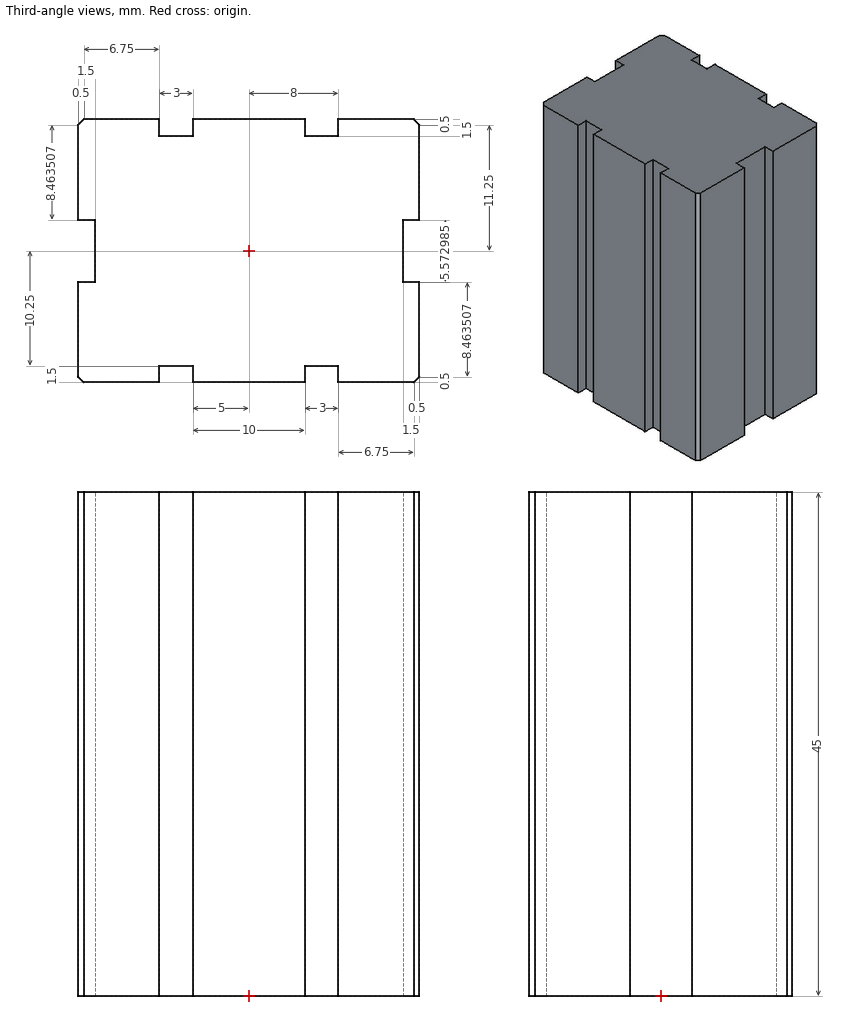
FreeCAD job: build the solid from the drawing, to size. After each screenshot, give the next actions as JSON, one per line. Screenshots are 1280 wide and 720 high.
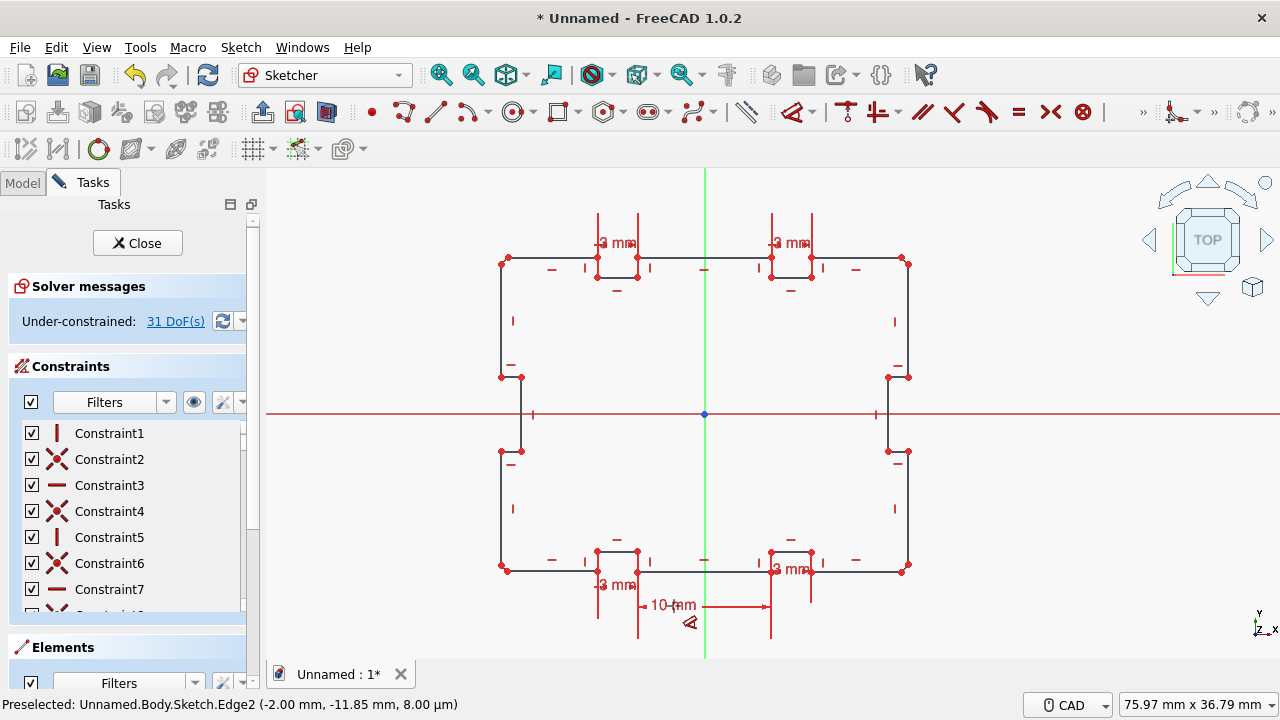
{"action": "left_click", "coordinate": [731, 258]}
{"action": "left_click", "coordinate": [674, 224]}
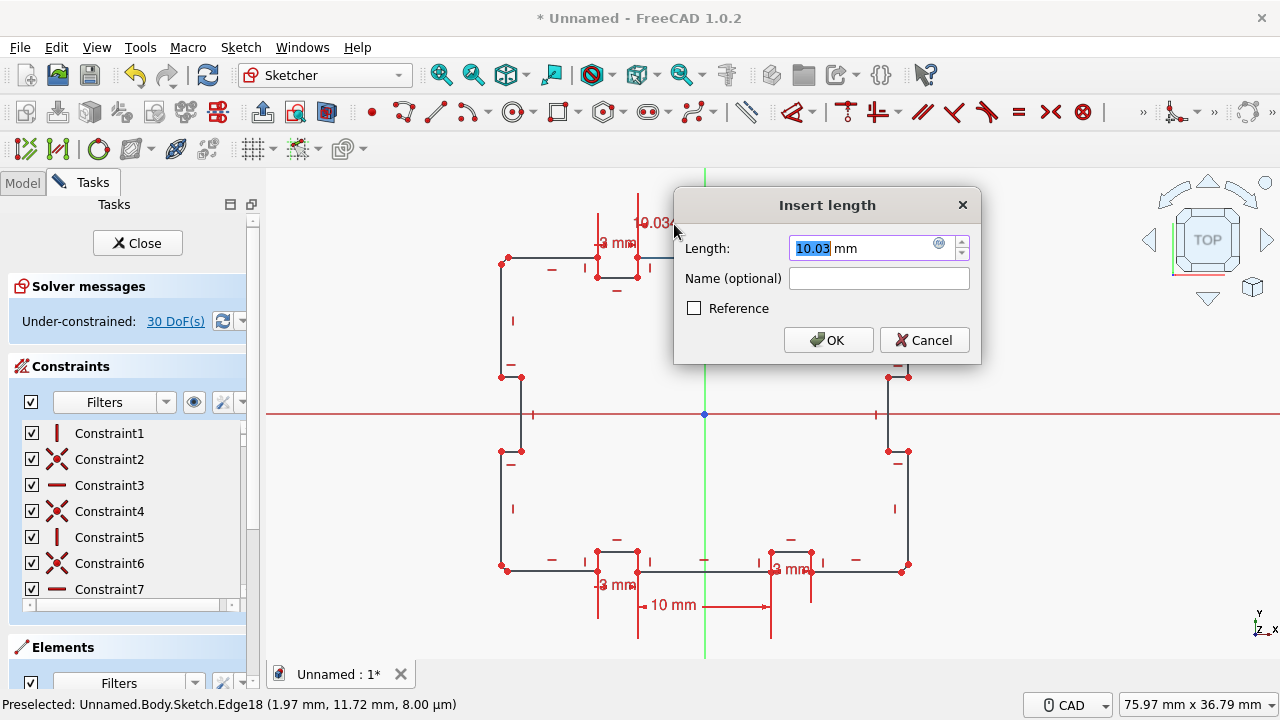
{"action": "type", "text": "10"}
{"action": "key", "text": "Return"}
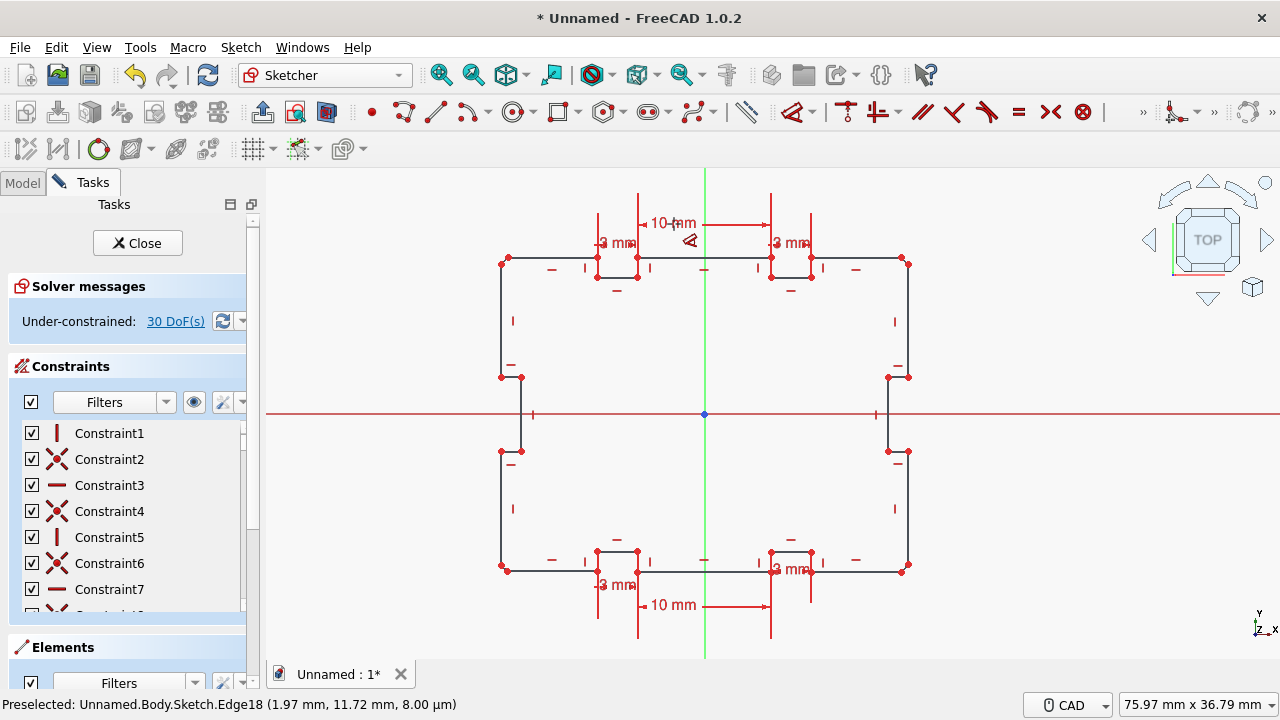
{"action": "left_click", "coordinate": [638, 552]}
{"action": "left_click", "coordinate": [671, 380]}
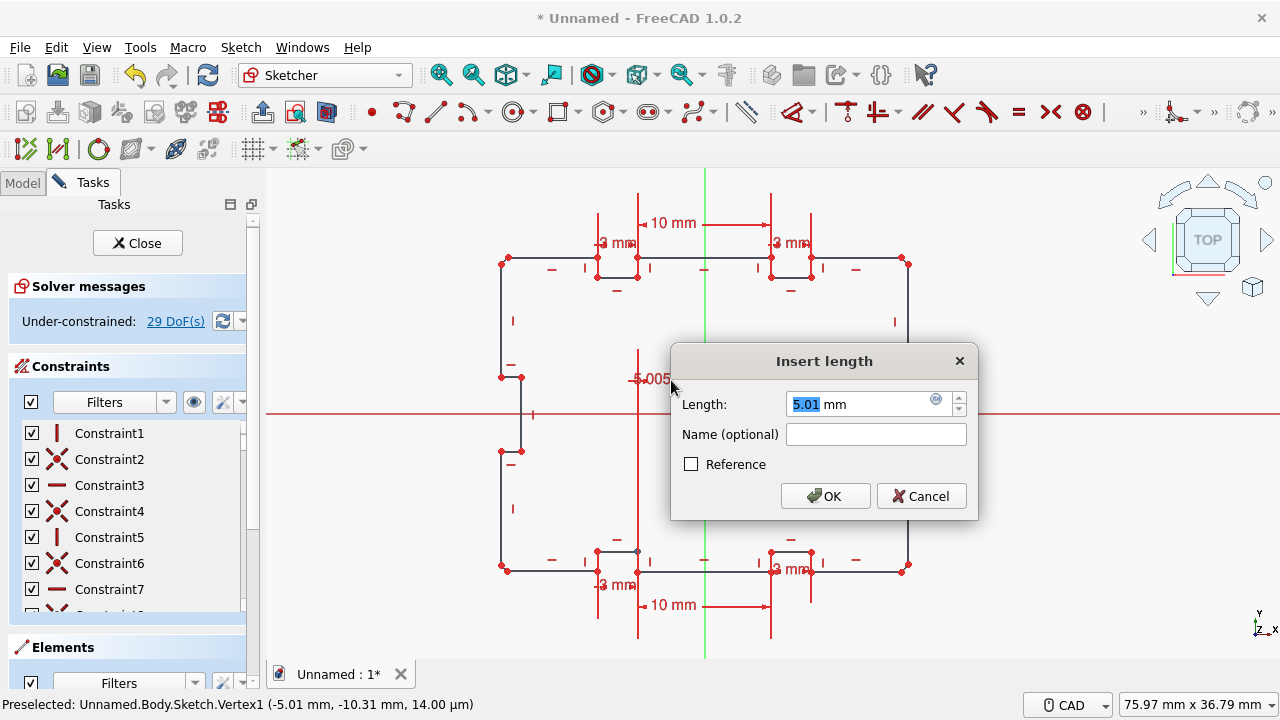
{"action": "type", "text": "5"}
{"action": "key", "text": "Return"}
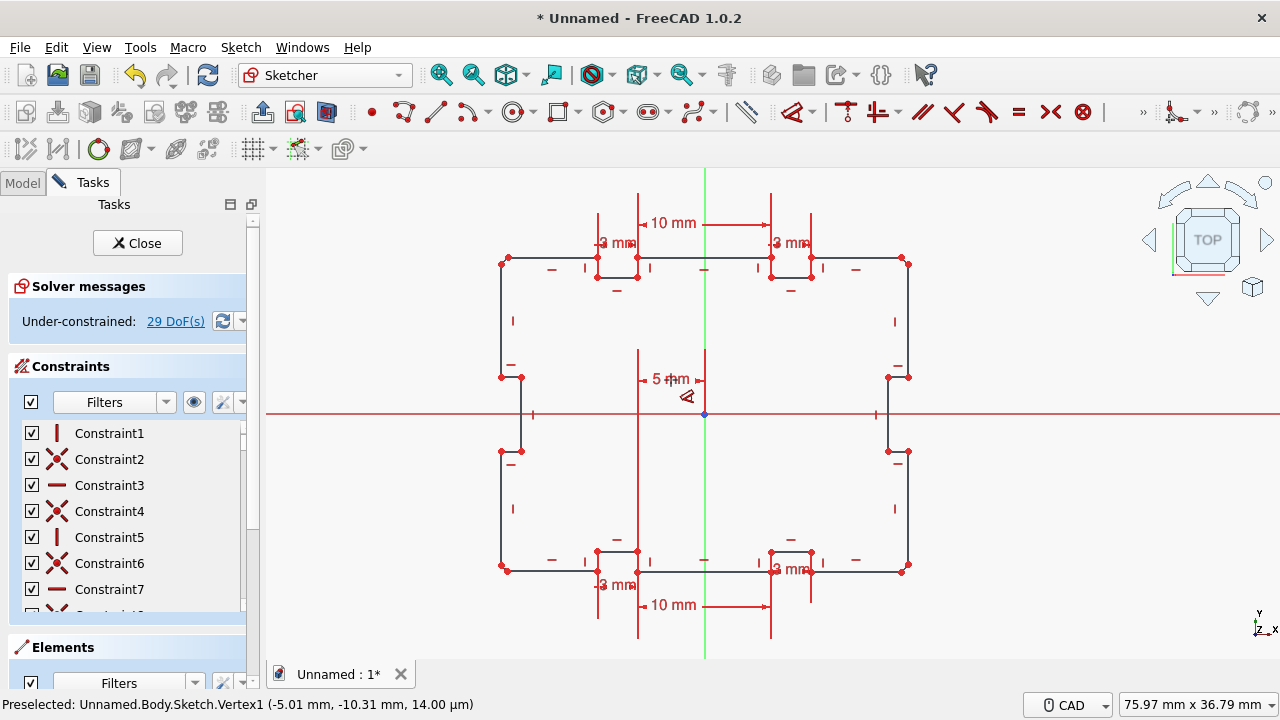
{"action": "left_click", "coordinate": [811, 258]}
{"action": "left_click", "coordinate": [758, 224]}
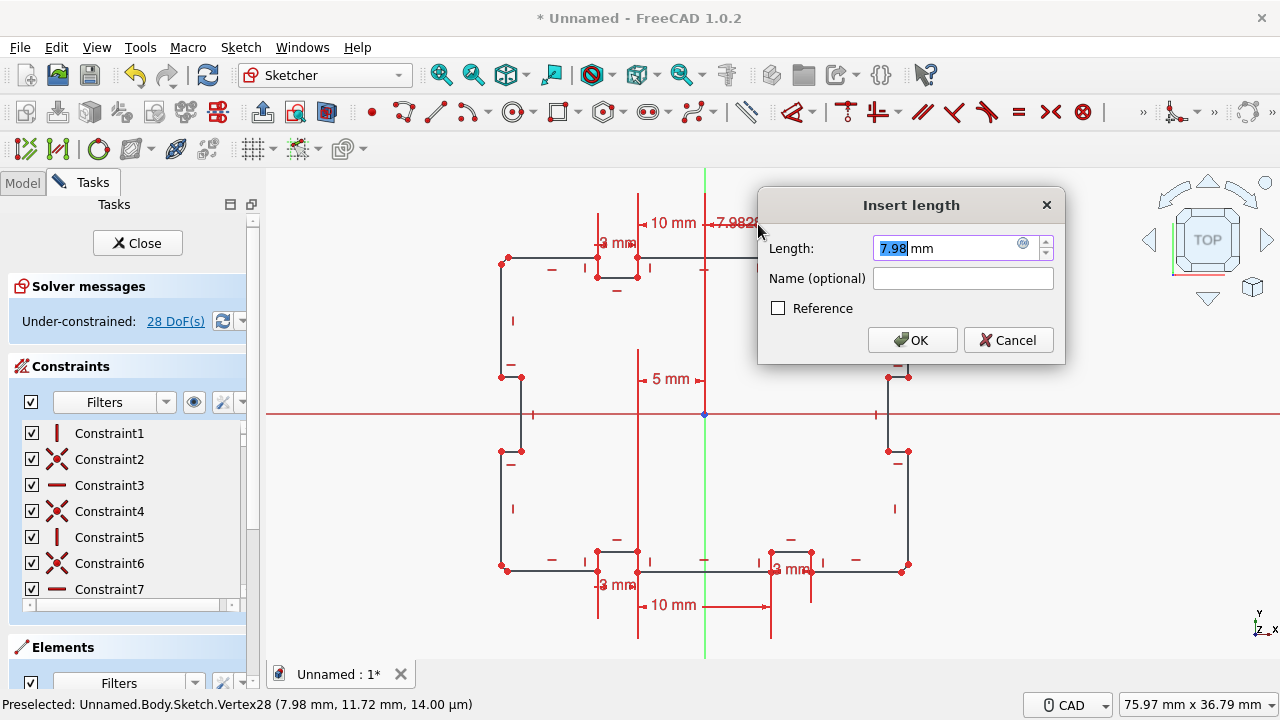
{"action": "type", "text": "8"}
{"action": "key", "text": "Return"}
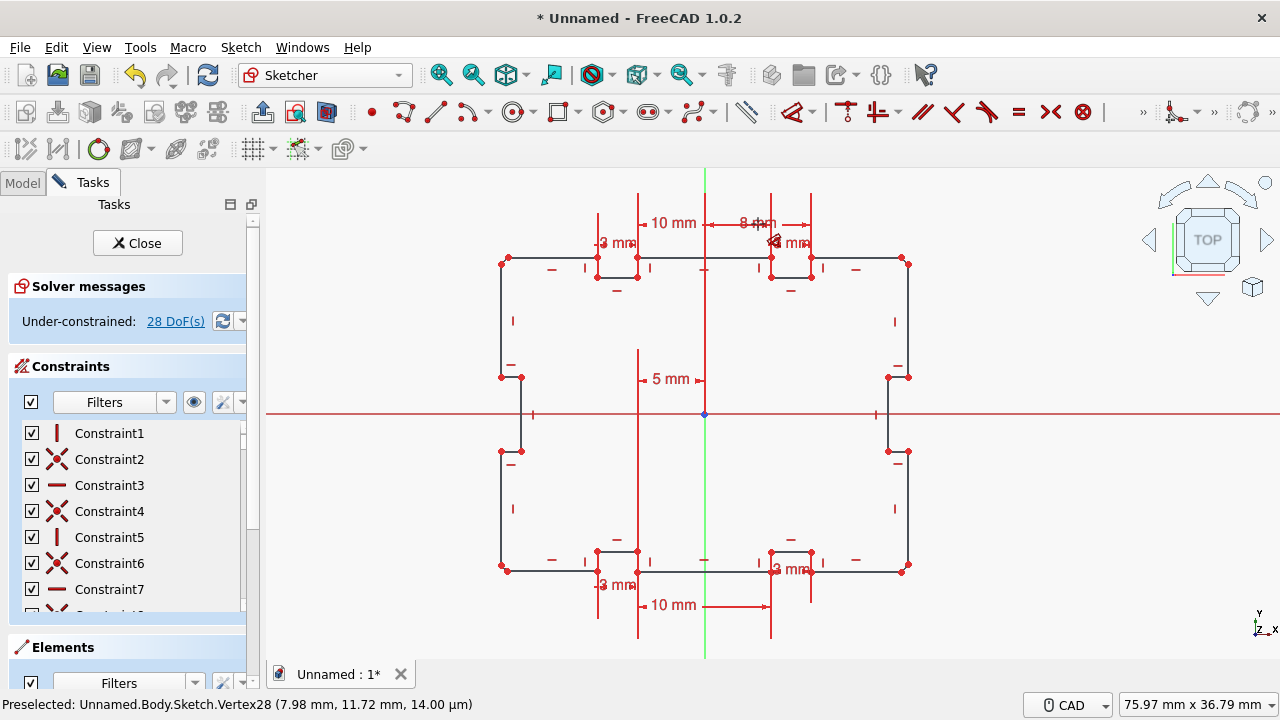
{"action": "scroll", "coordinate": [638, 562], "scroll_direction": "up", "scroll_amount": 4}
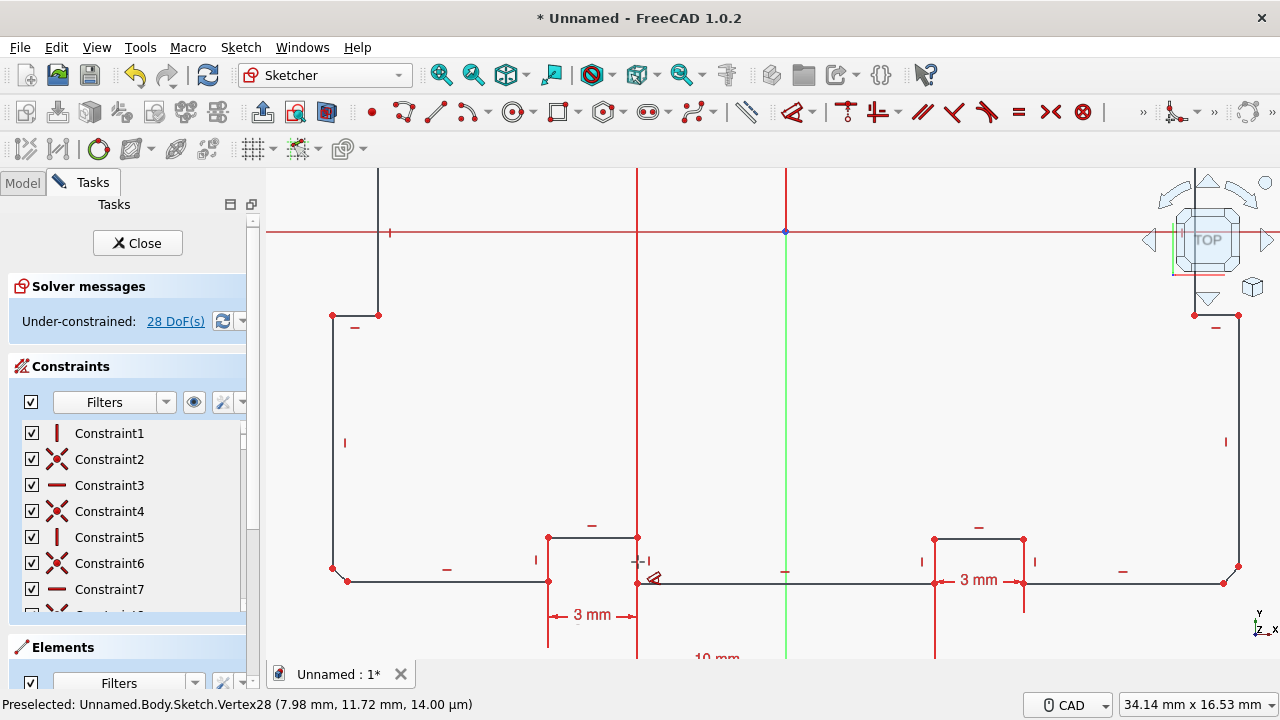
{"action": "left_click", "coordinate": [637, 561]}
{"action": "left_click", "coordinate": [603, 561]}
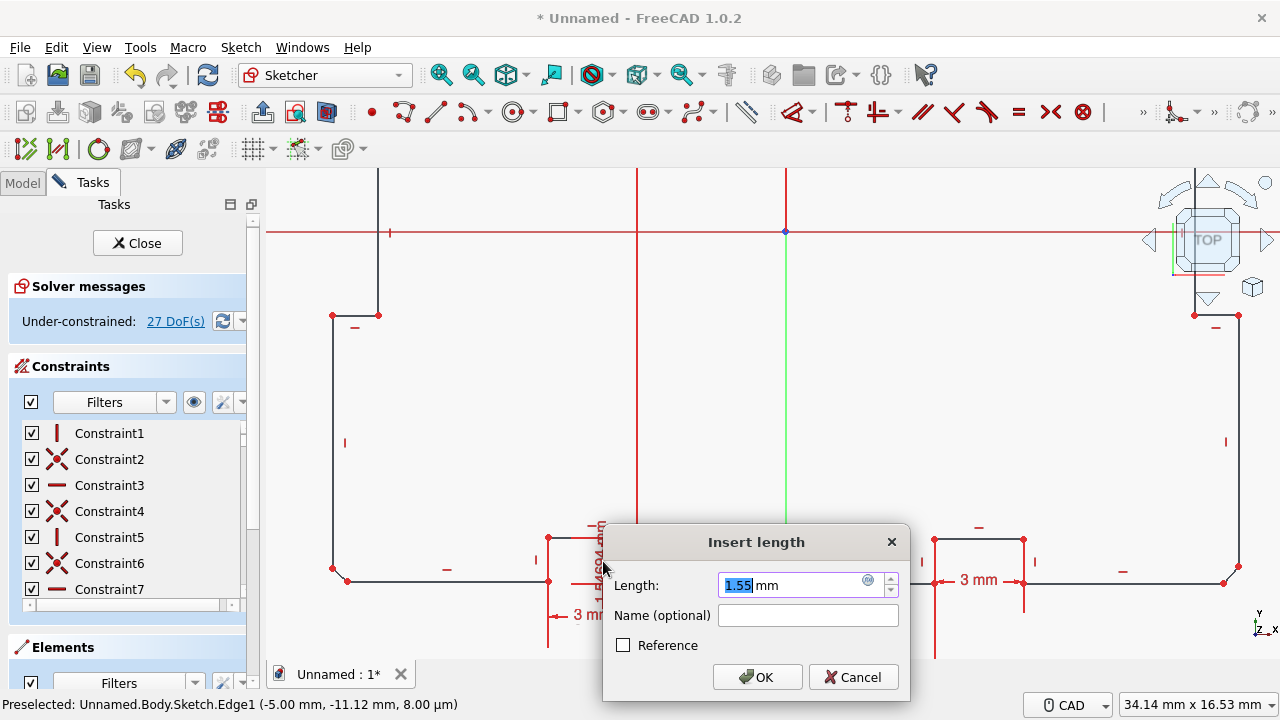
{"action": "type", "text": "1.5"}
{"action": "key", "text": "Return"}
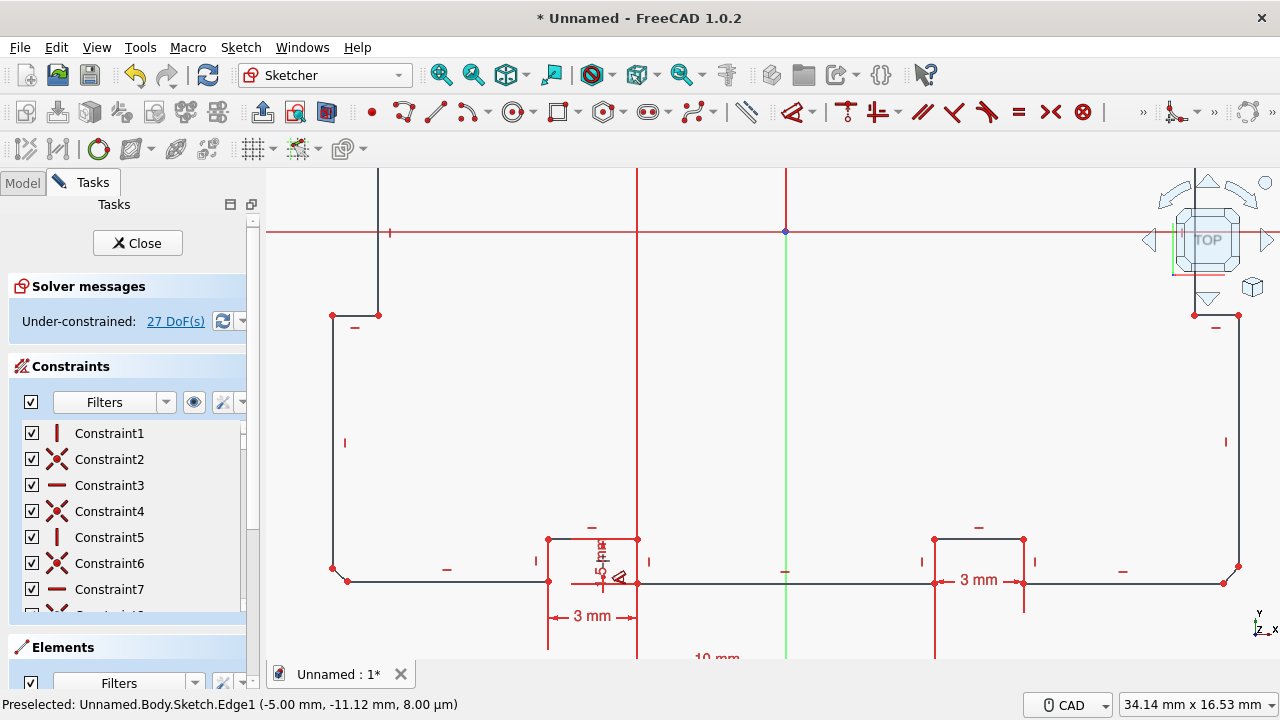
{"action": "left_click", "coordinate": [935, 570]}
{"action": "left_click", "coordinate": [901, 562]}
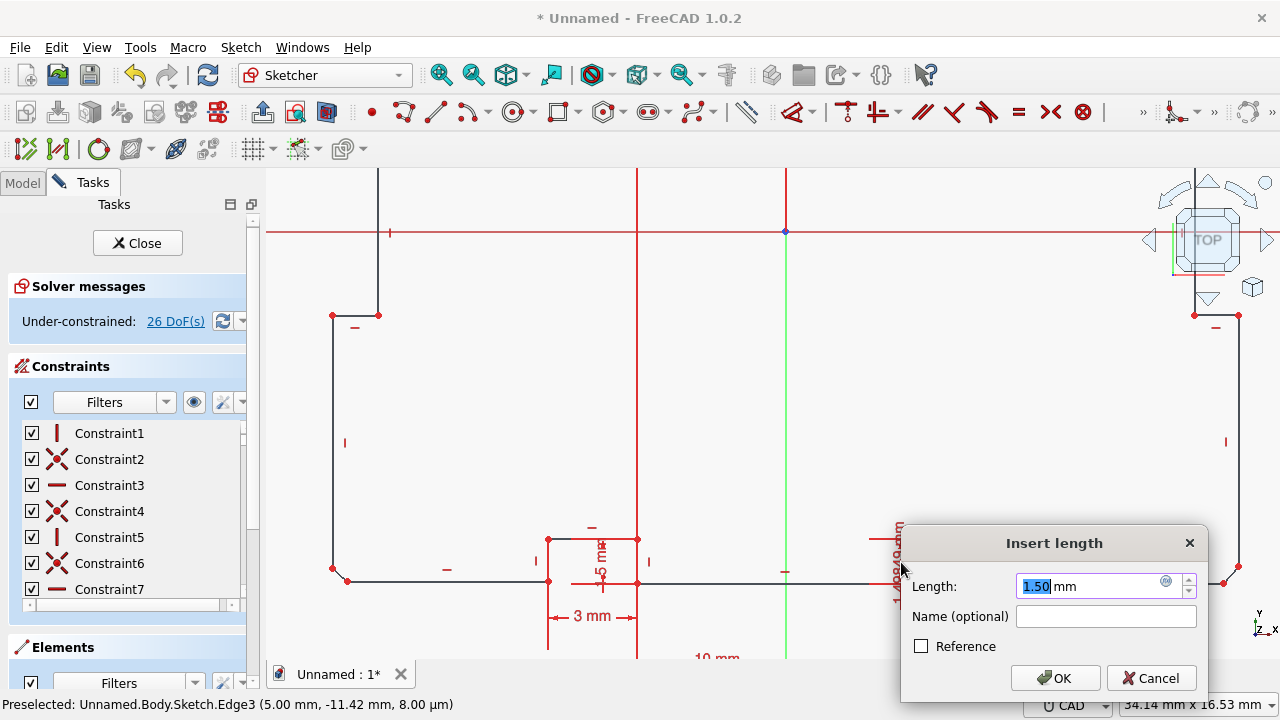
{"action": "type", "text": "1.5"}
{"action": "key", "text": "Return"}